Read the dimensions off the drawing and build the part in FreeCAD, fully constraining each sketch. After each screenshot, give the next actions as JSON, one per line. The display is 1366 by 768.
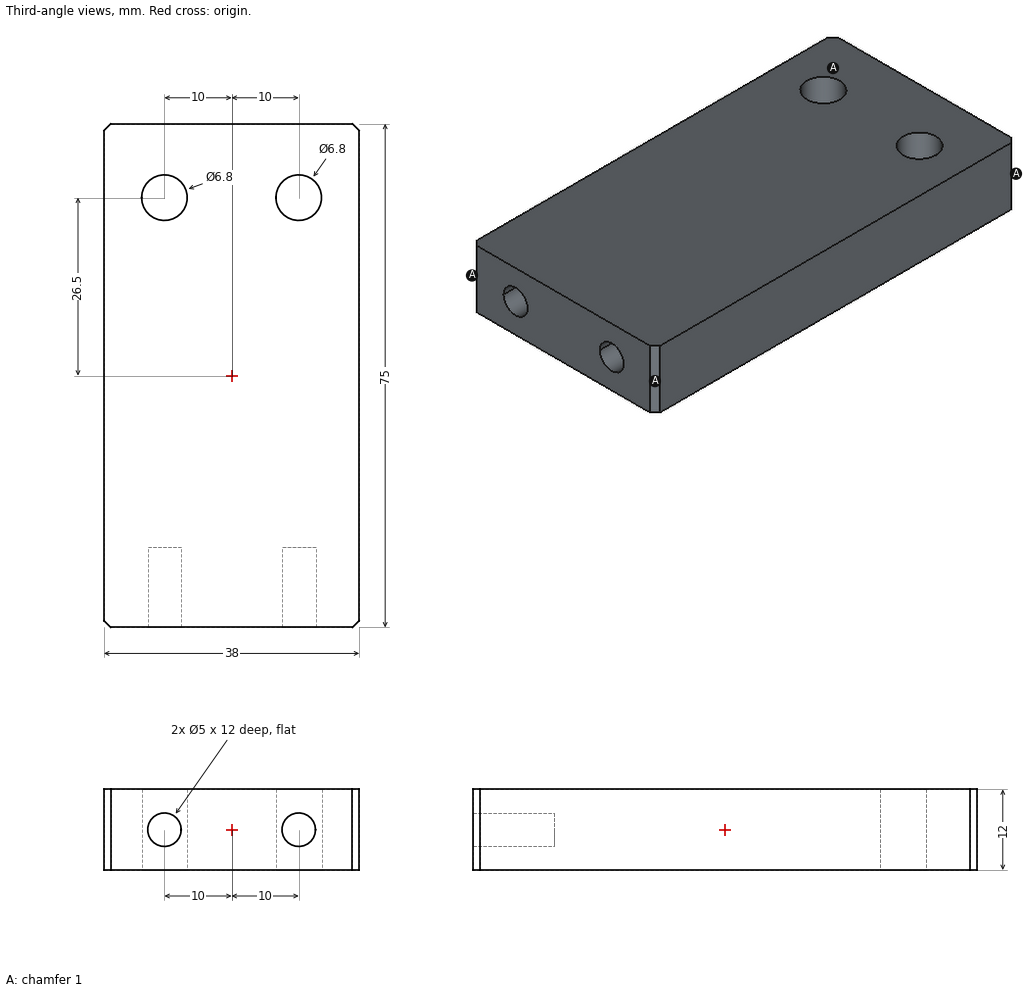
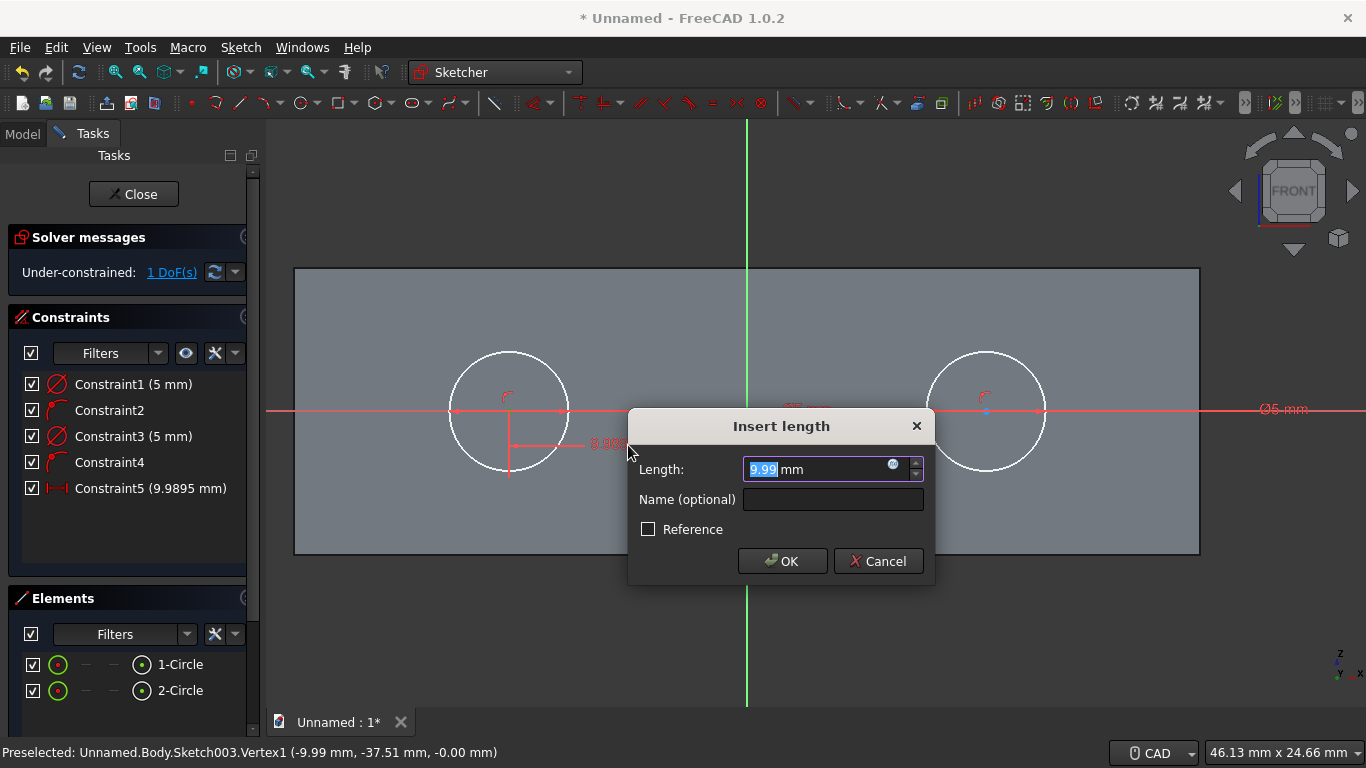
{"action": "type", "text": "10"}
{"action": "key", "text": "Return"}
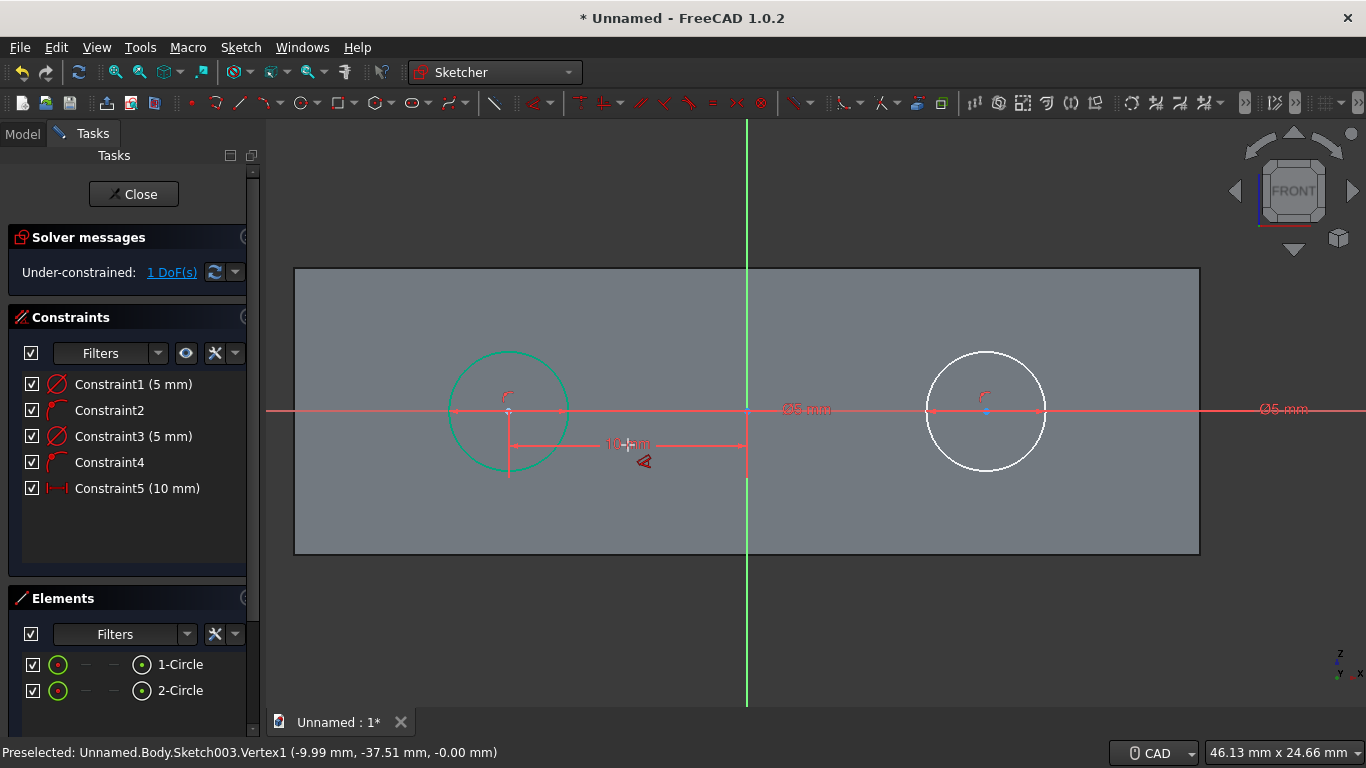
{"action": "left_click", "coordinate": [986, 411]}
{"action": "left_click", "coordinate": [867, 445]}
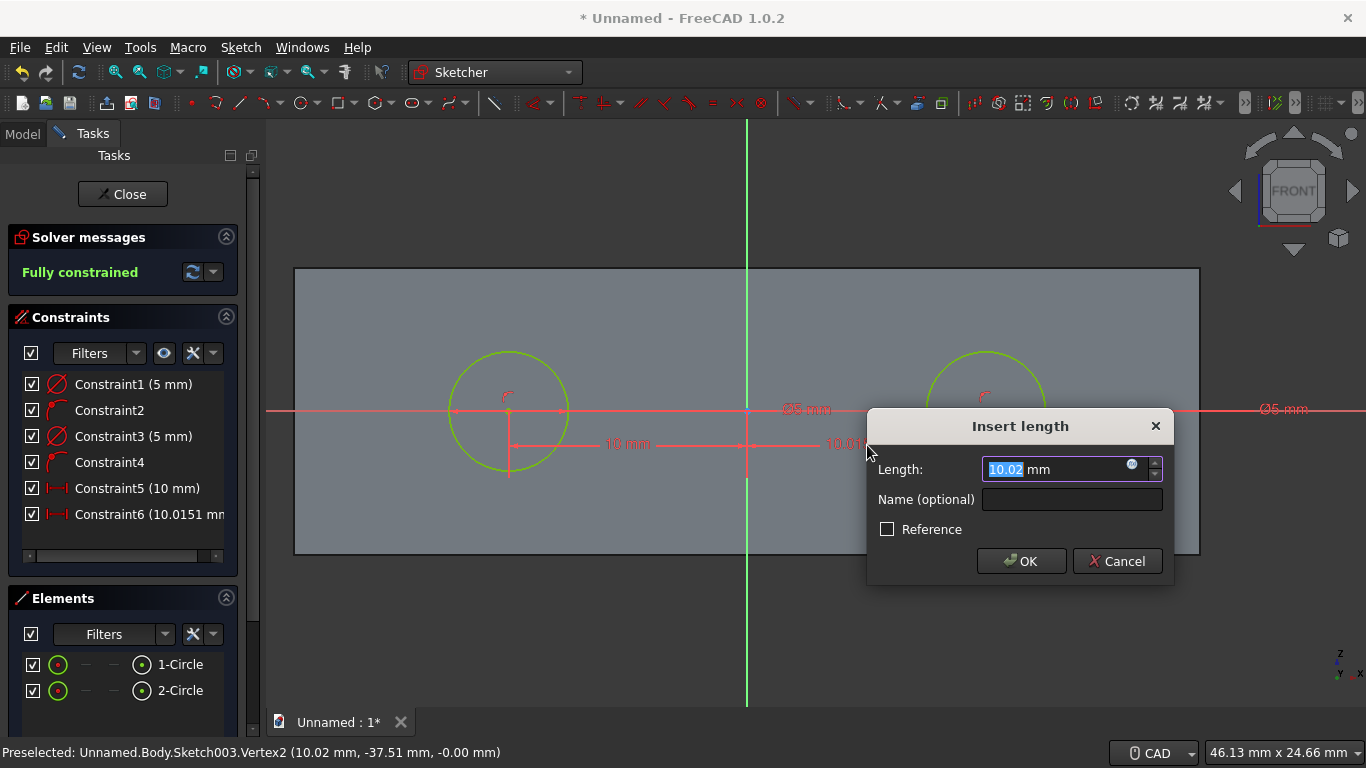
{"action": "type", "text": "10"}
{"action": "key", "text": "Return"}
{"action": "key", "text": "Escape"}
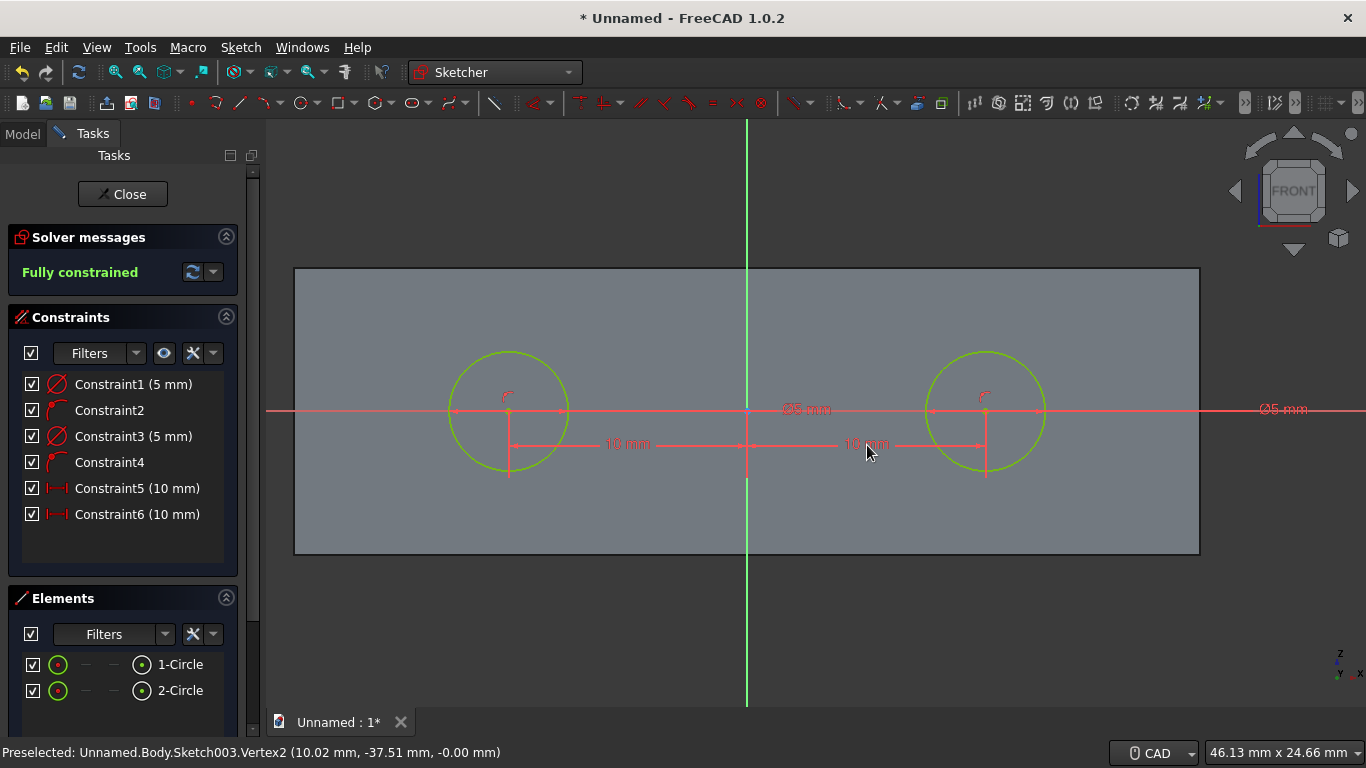
{"action": "left_click", "coordinate": [123, 194]}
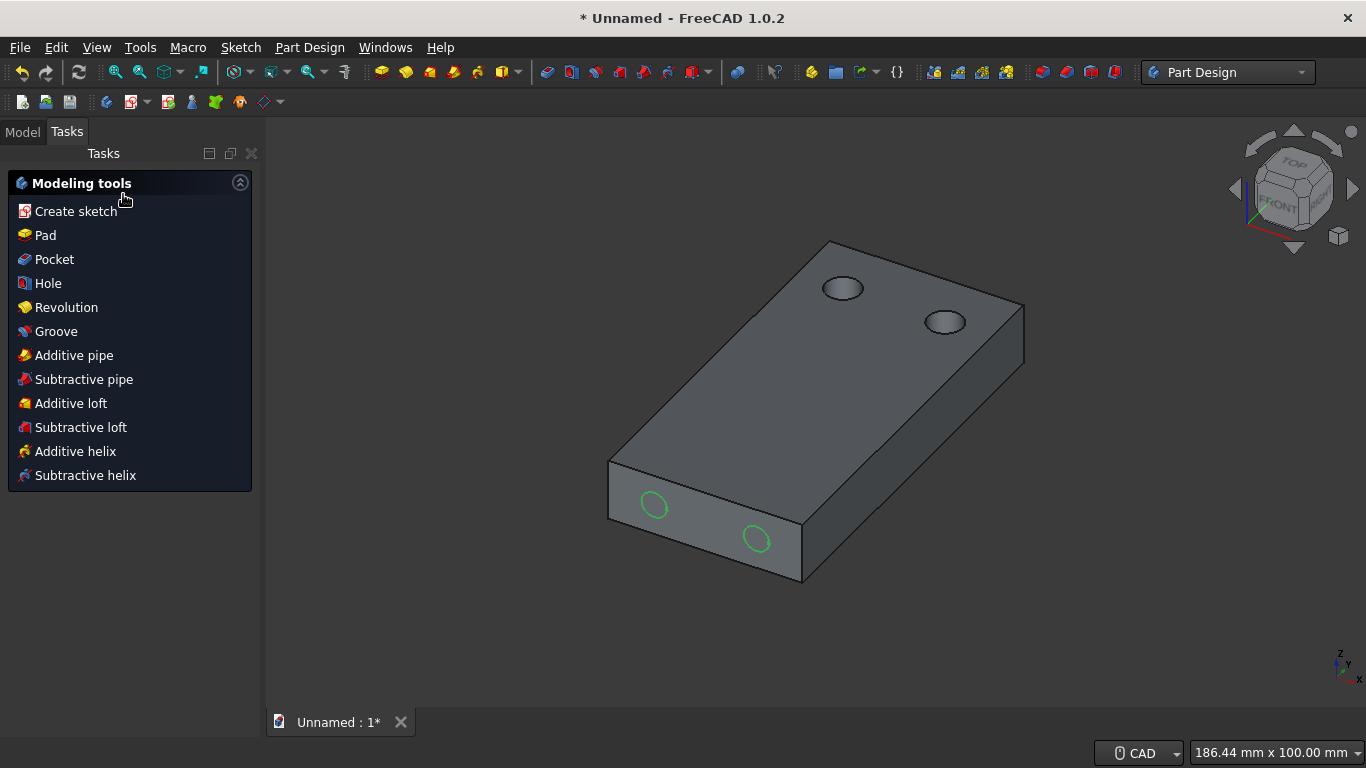
{"action": "left_click", "coordinate": [572, 72]}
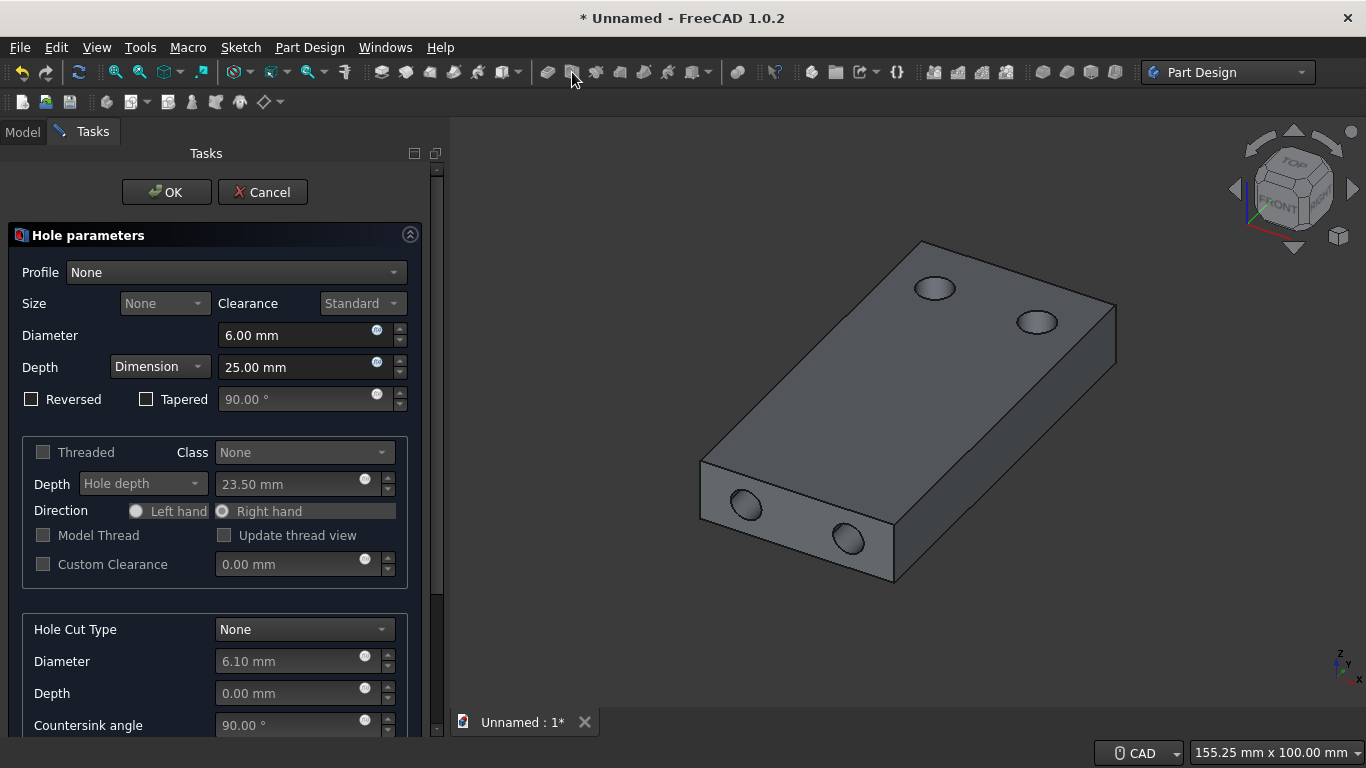
{"action": "triple_click", "coordinate": [305, 335]}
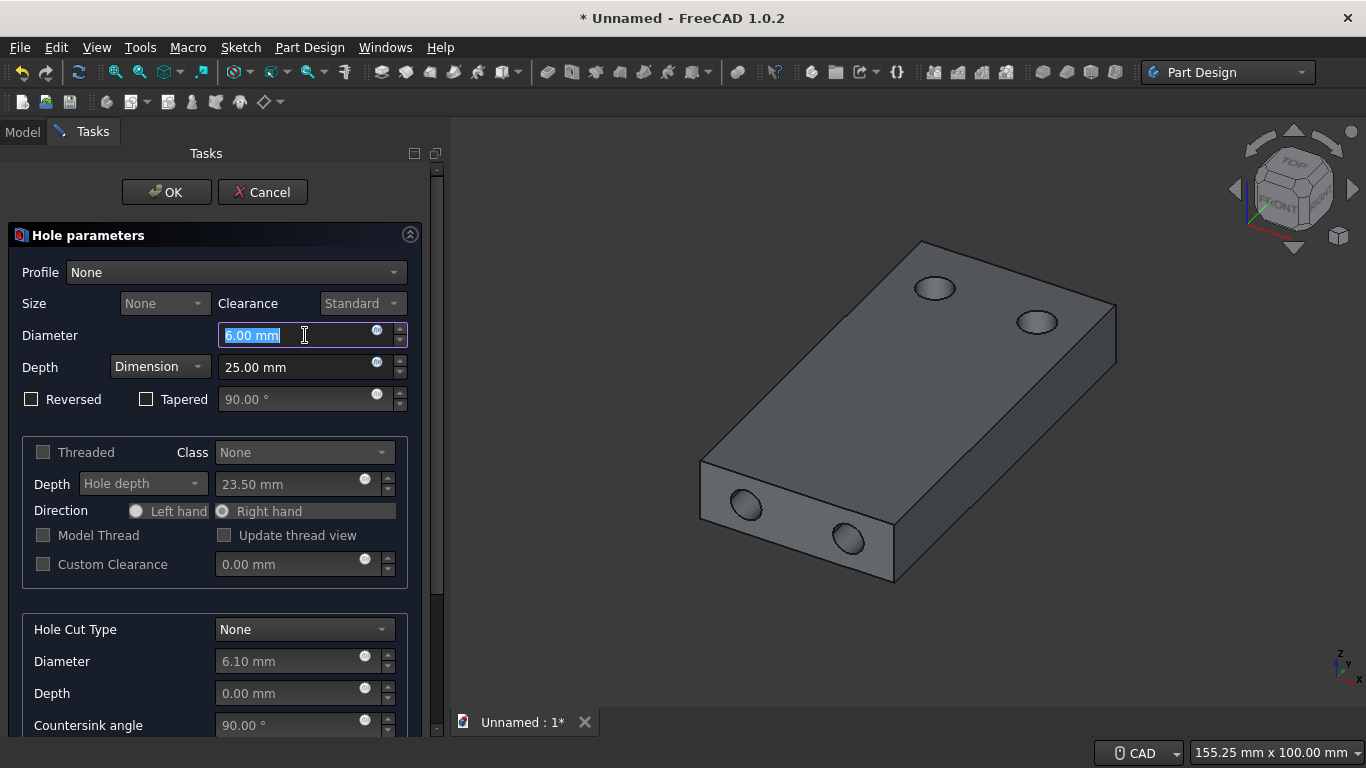
{"action": "type", "text": "5"}
{"action": "key", "text": "Tab"}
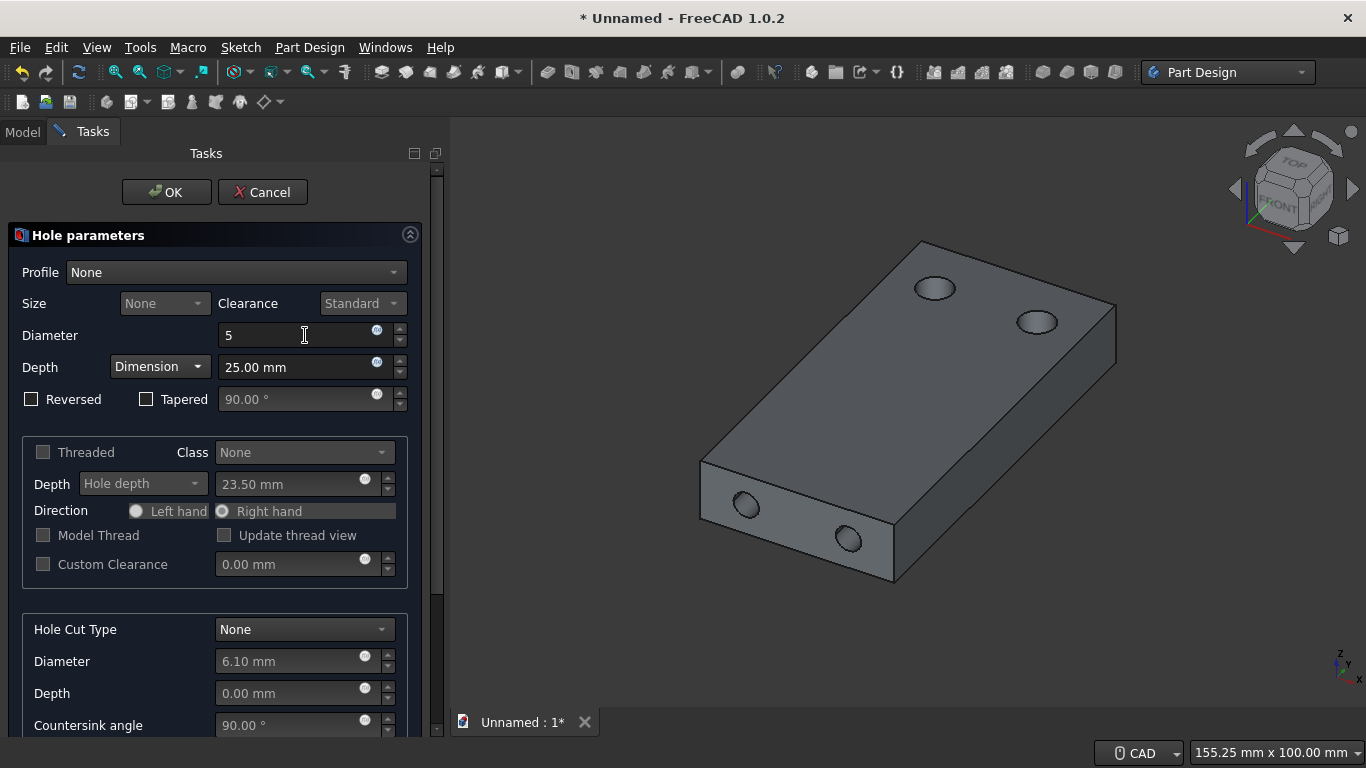
{"action": "triple_click", "coordinate": [305, 367]}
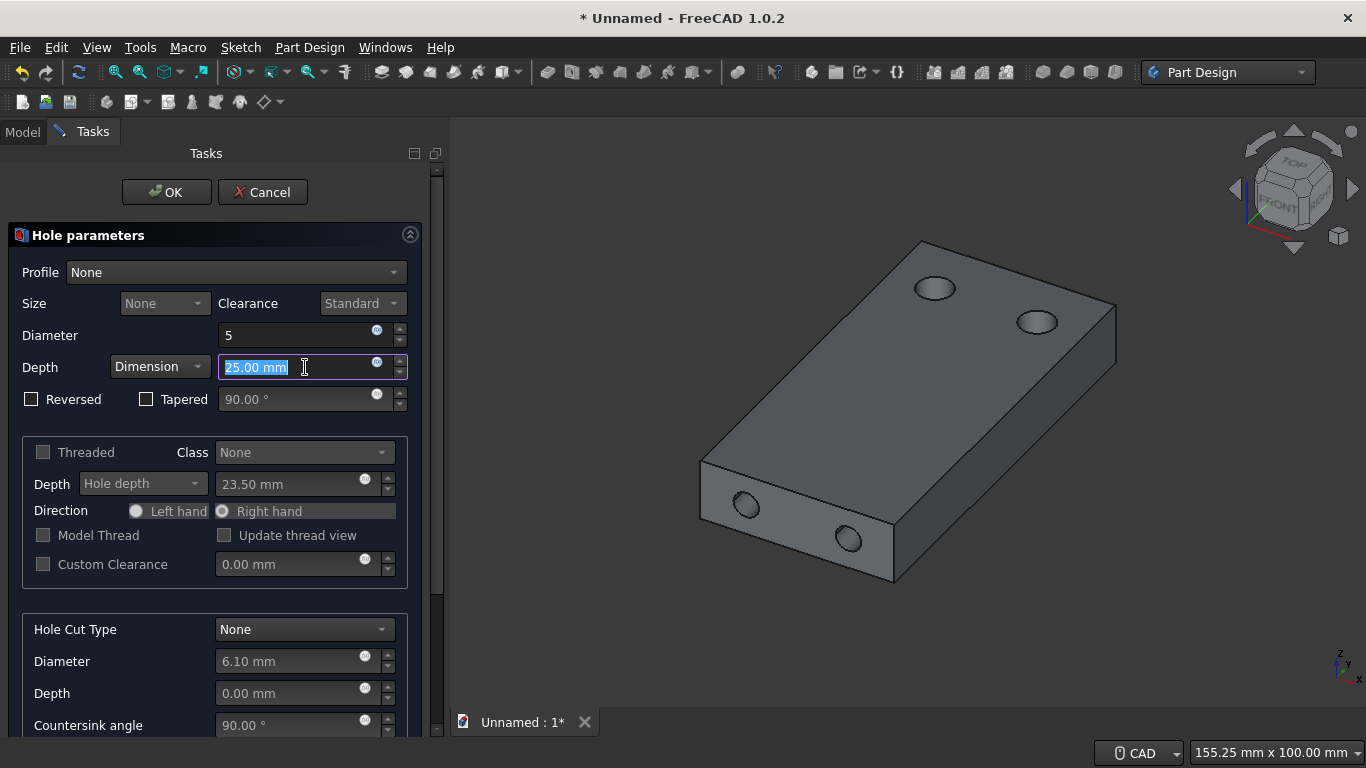
{"action": "type", "text": "12"}
{"action": "key", "text": "Tab"}